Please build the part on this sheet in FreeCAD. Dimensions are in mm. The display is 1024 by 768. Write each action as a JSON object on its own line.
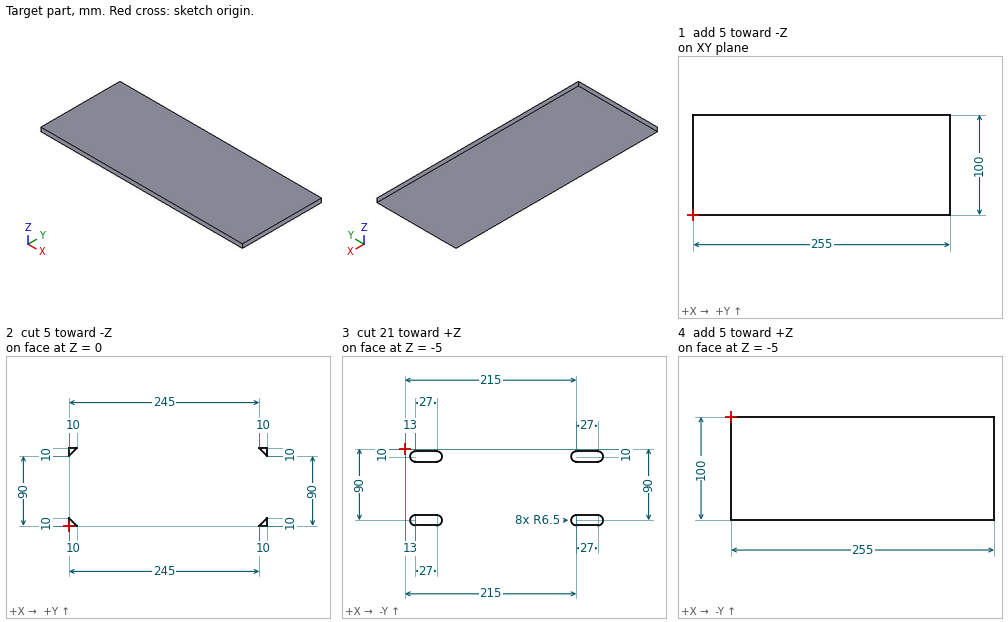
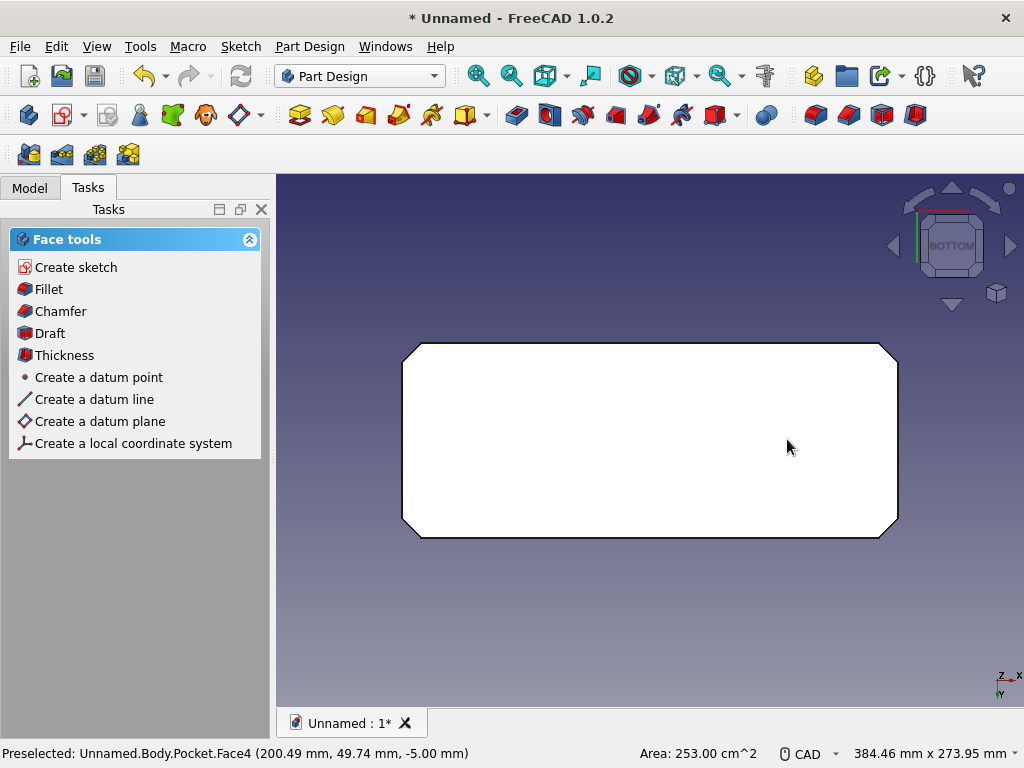
{"action": "left_click", "coordinate": [62, 116]}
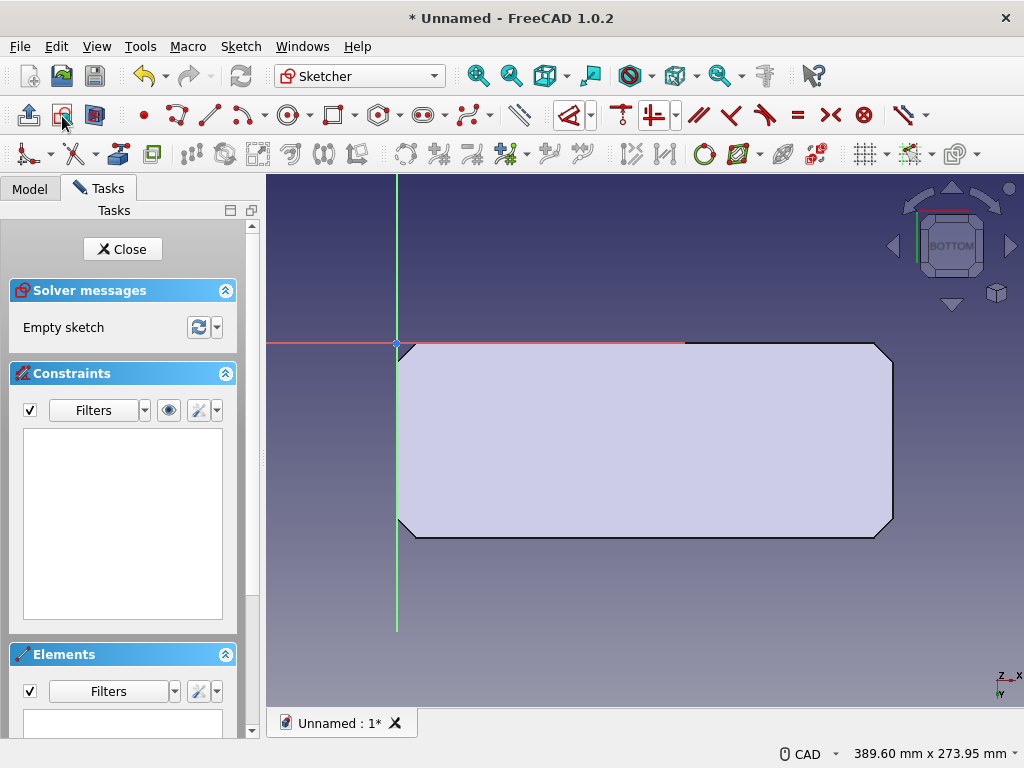
{"action": "scroll", "coordinate": [296, 456], "scroll_direction": "down", "scroll_amount": 1}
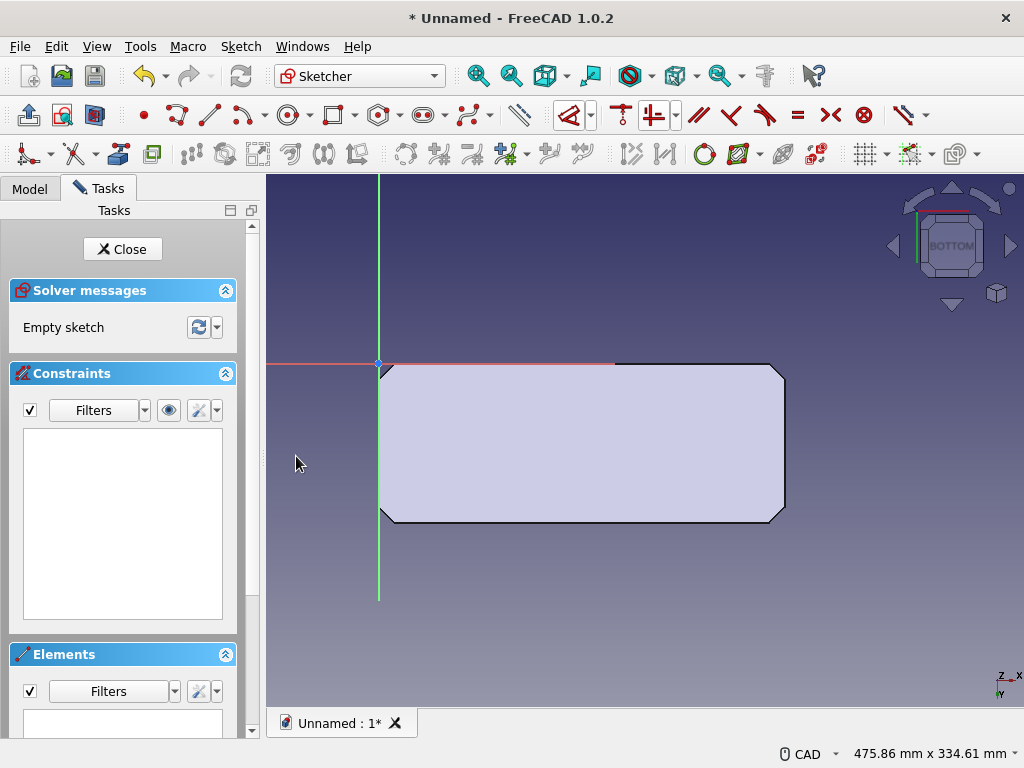
{"action": "key", "text": "g s"}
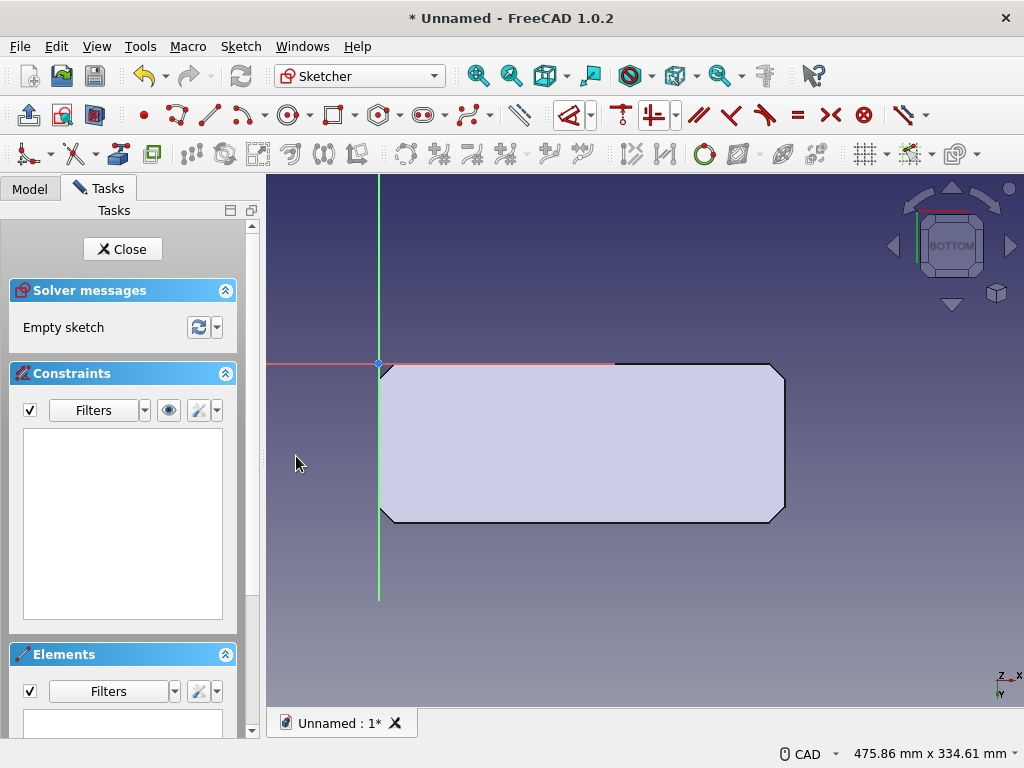
{"action": "scroll", "coordinate": [721, 507], "scroll_direction": "up", "scroll_amount": 4}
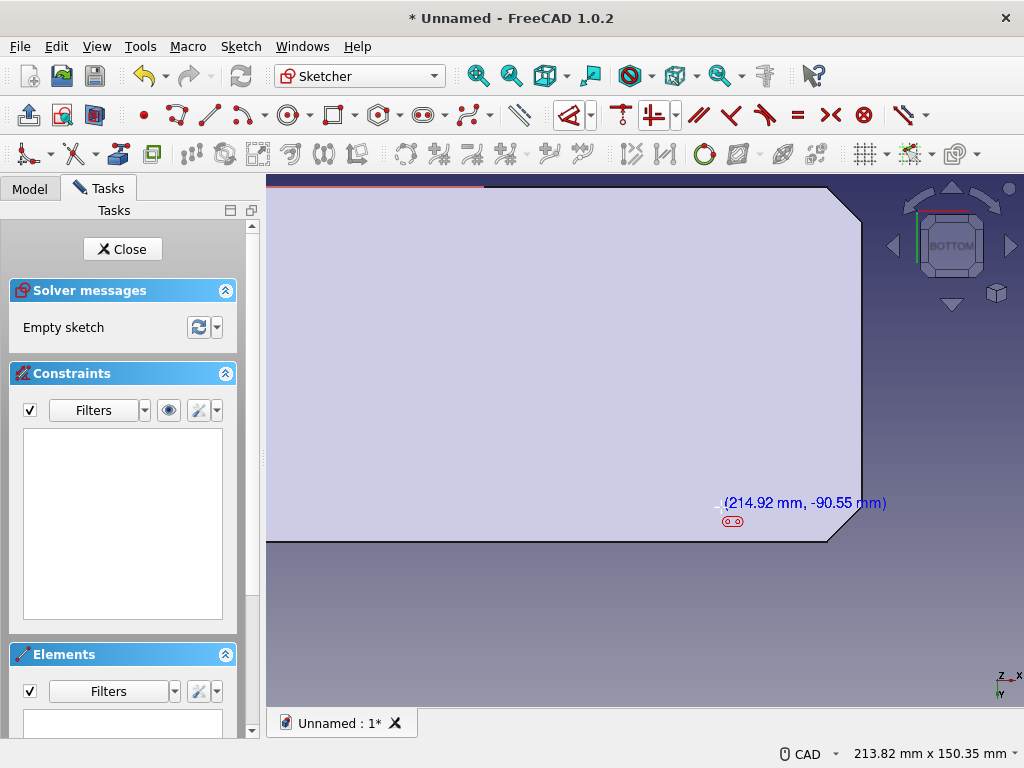
{"action": "left_click", "coordinate": [721, 507]}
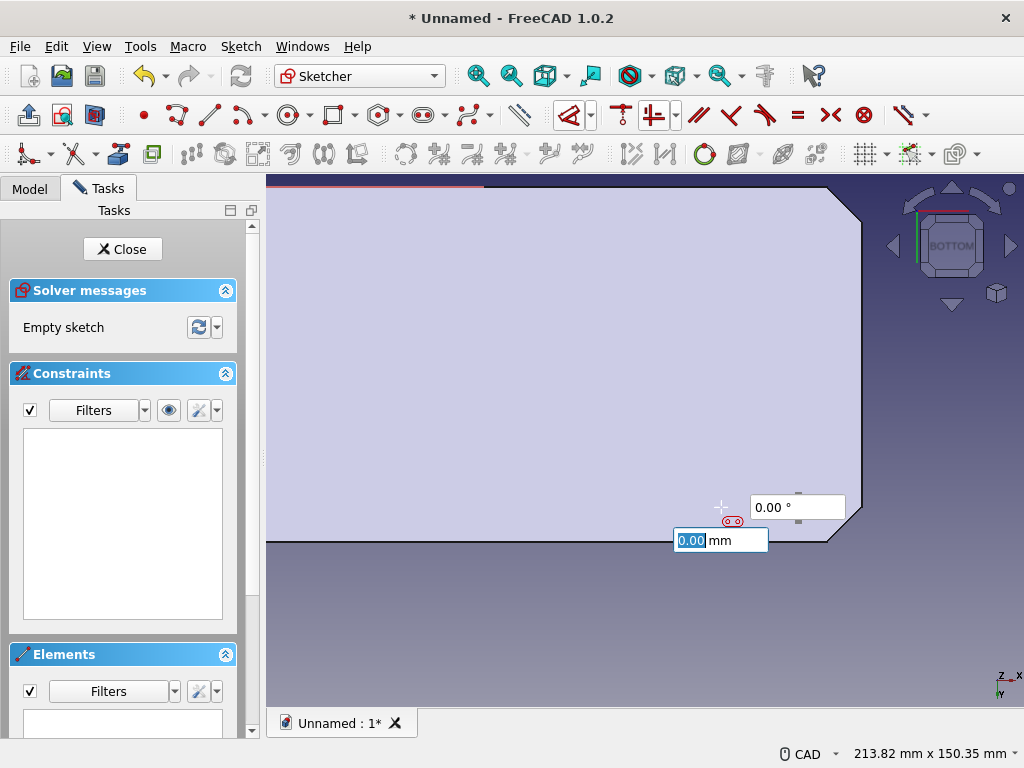
{"action": "left_click", "coordinate": [816, 507]}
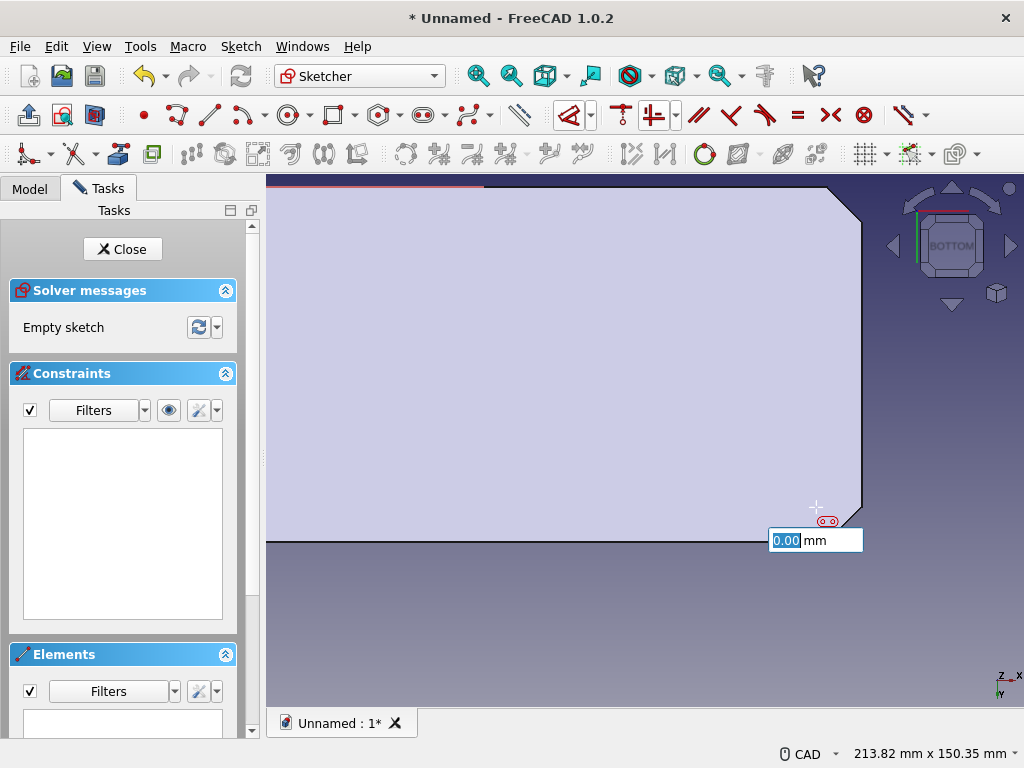
{"action": "left_click", "coordinate": [768, 483]}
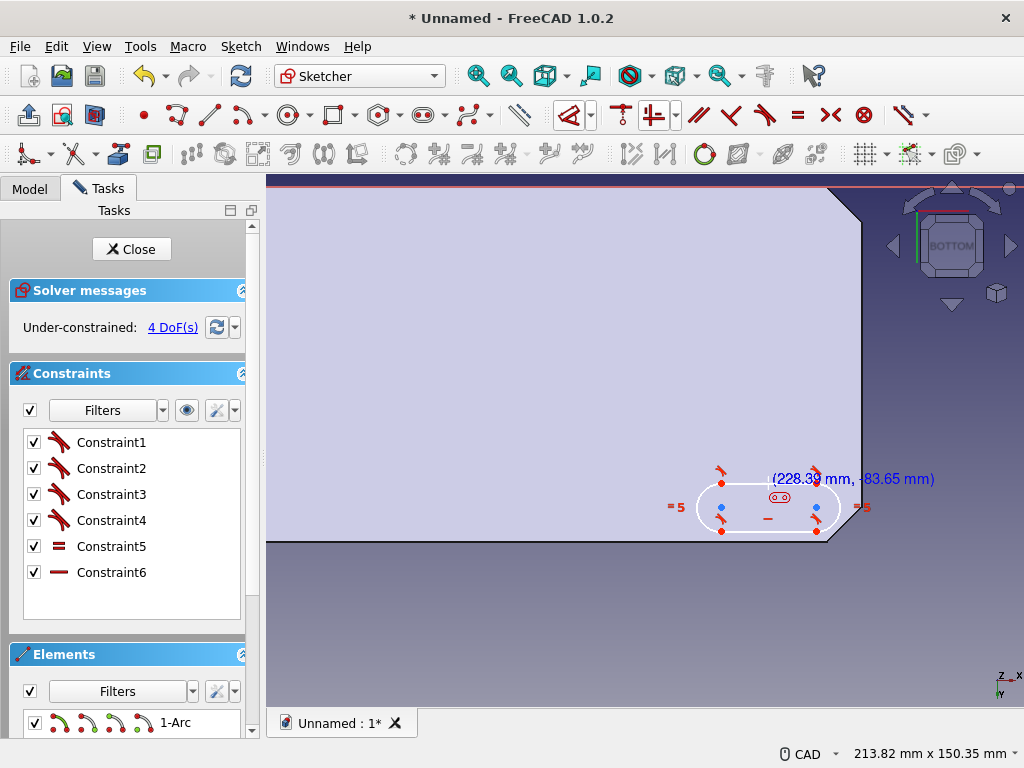
{"action": "scroll", "coordinate": [721, 507], "scroll_direction": "down", "scroll_amount": 4}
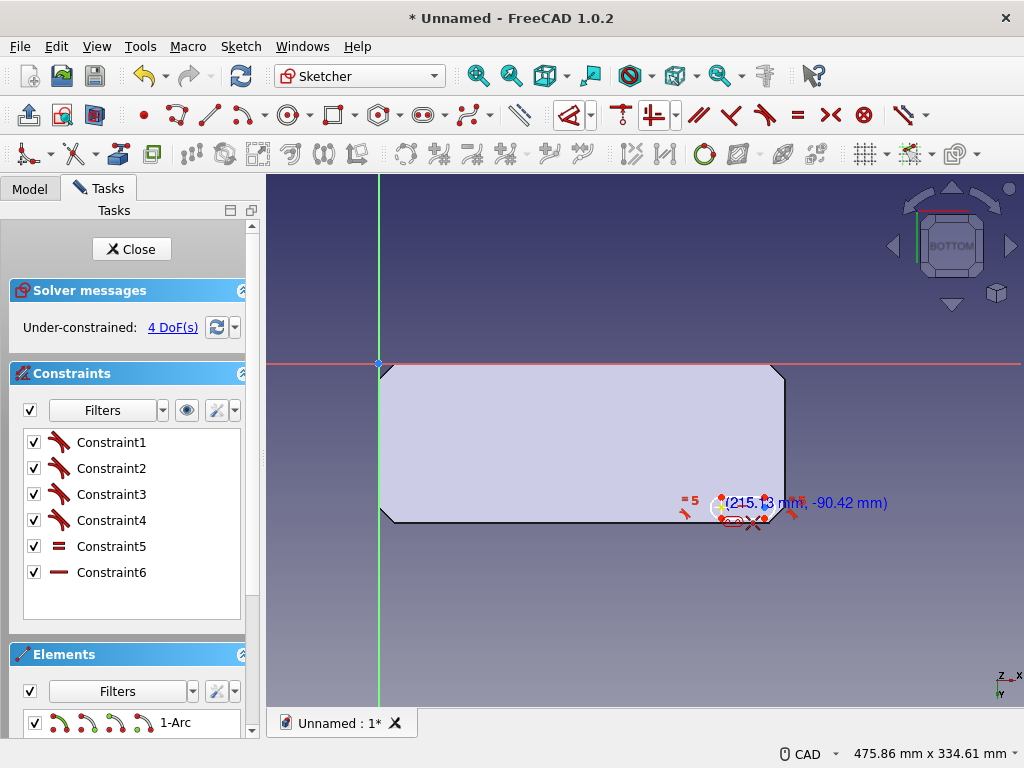
{"action": "scroll", "coordinate": [399, 507], "scroll_direction": "up", "scroll_amount": 4}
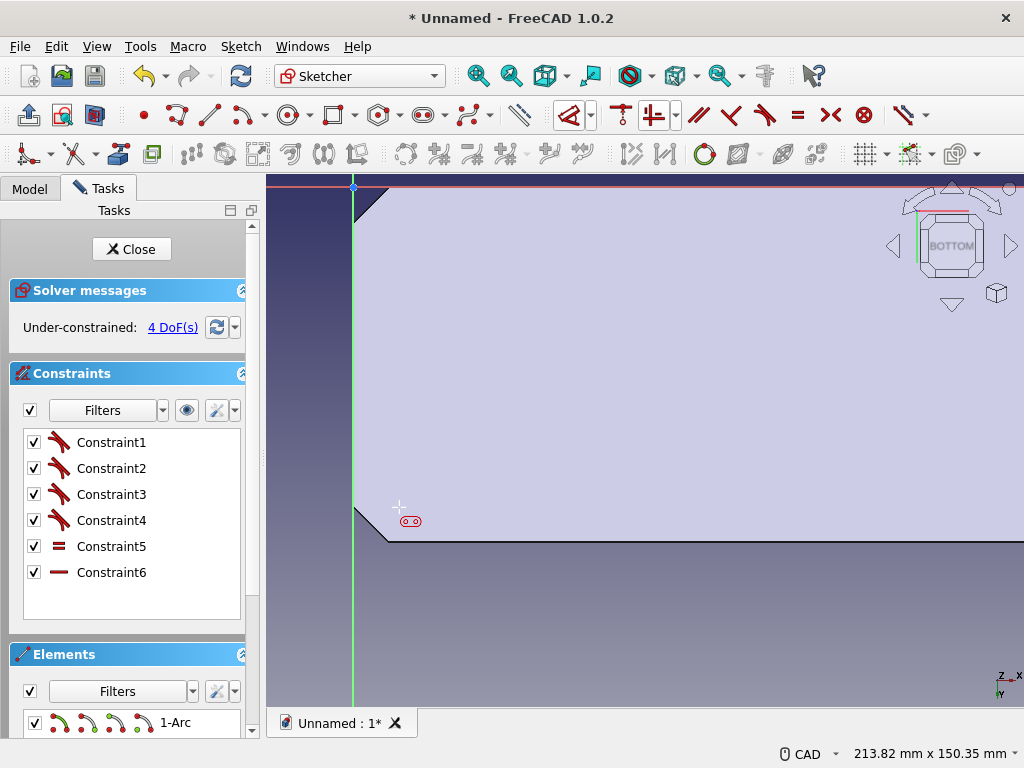
{"action": "left_click", "coordinate": [400, 507]}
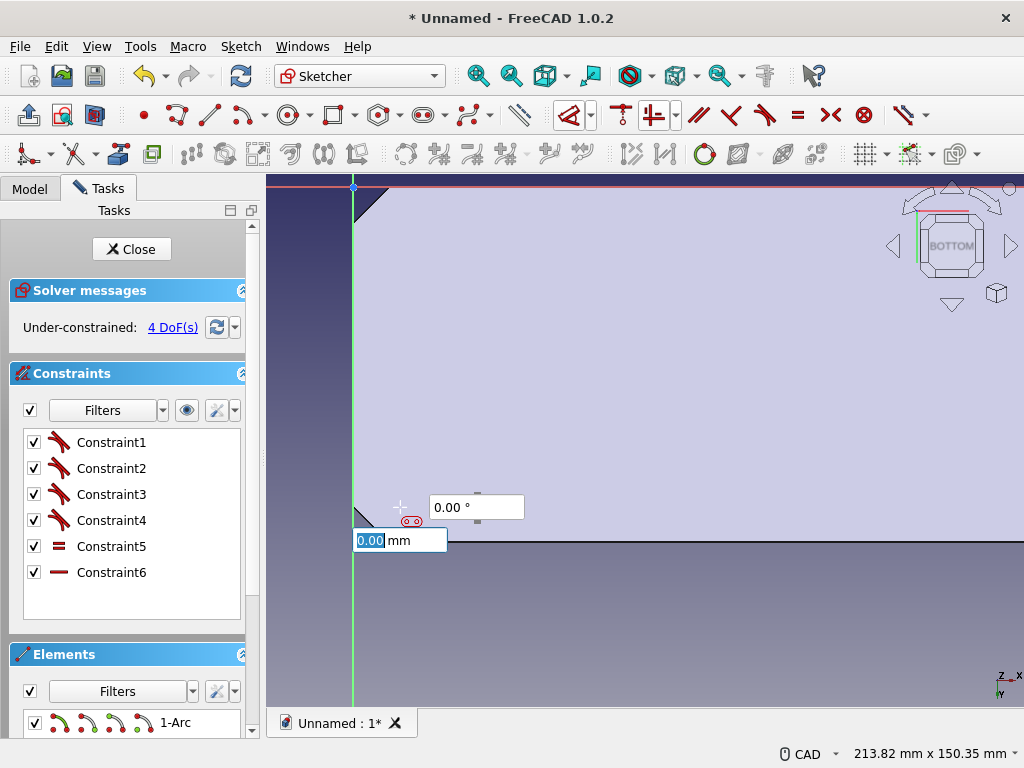
{"action": "left_click", "coordinate": [495, 507]}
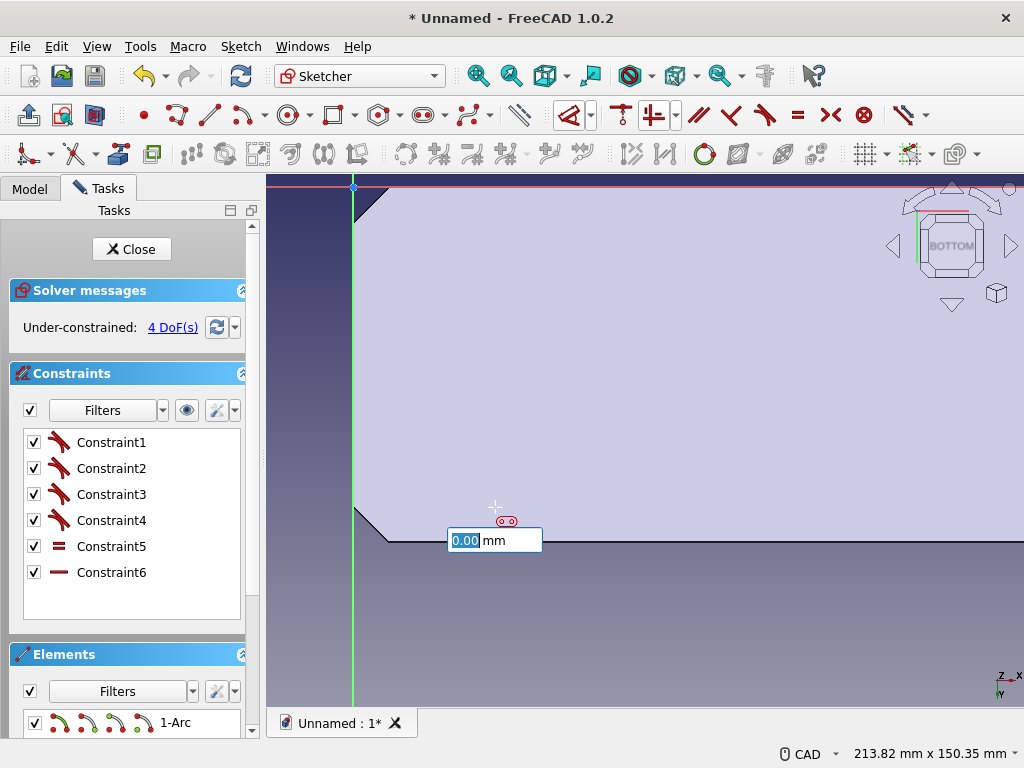
{"action": "left_click", "coordinate": [447, 530]}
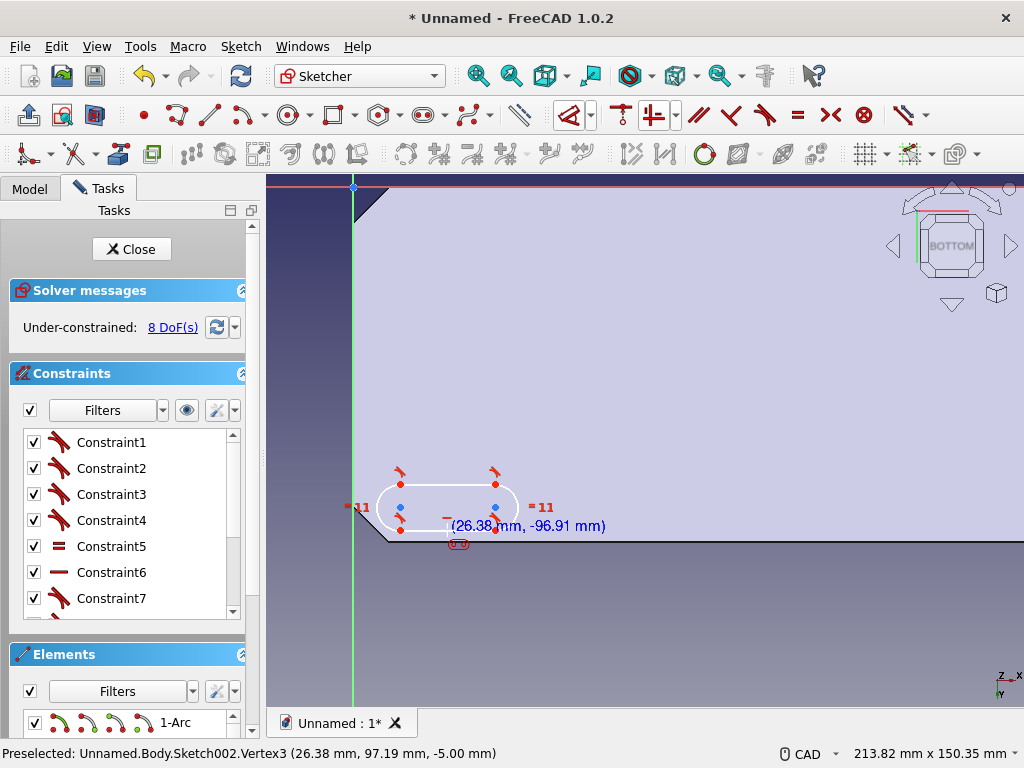
{"action": "left_click", "coordinate": [400, 223]}